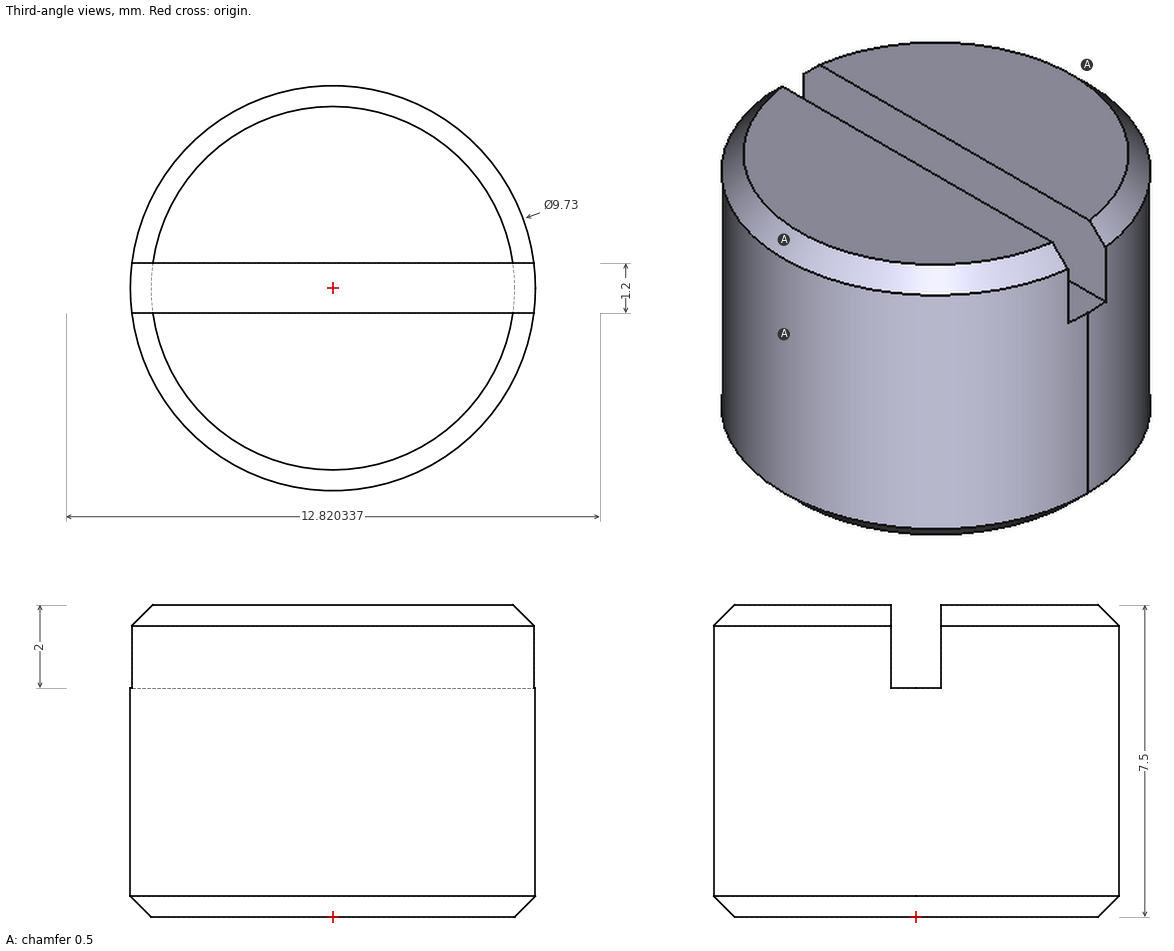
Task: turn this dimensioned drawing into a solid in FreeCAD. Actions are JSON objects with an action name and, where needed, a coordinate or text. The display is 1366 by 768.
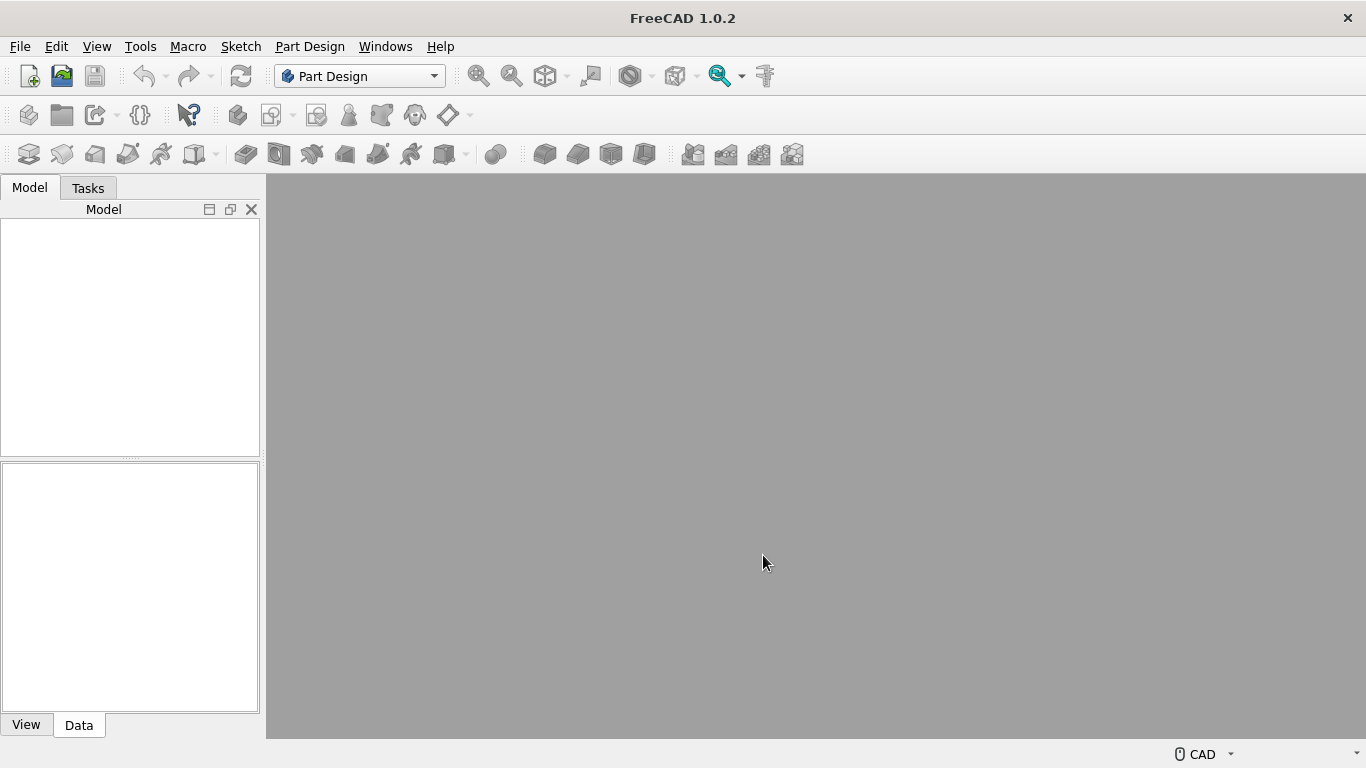
{"action": "left_click", "coordinate": [29, 76]}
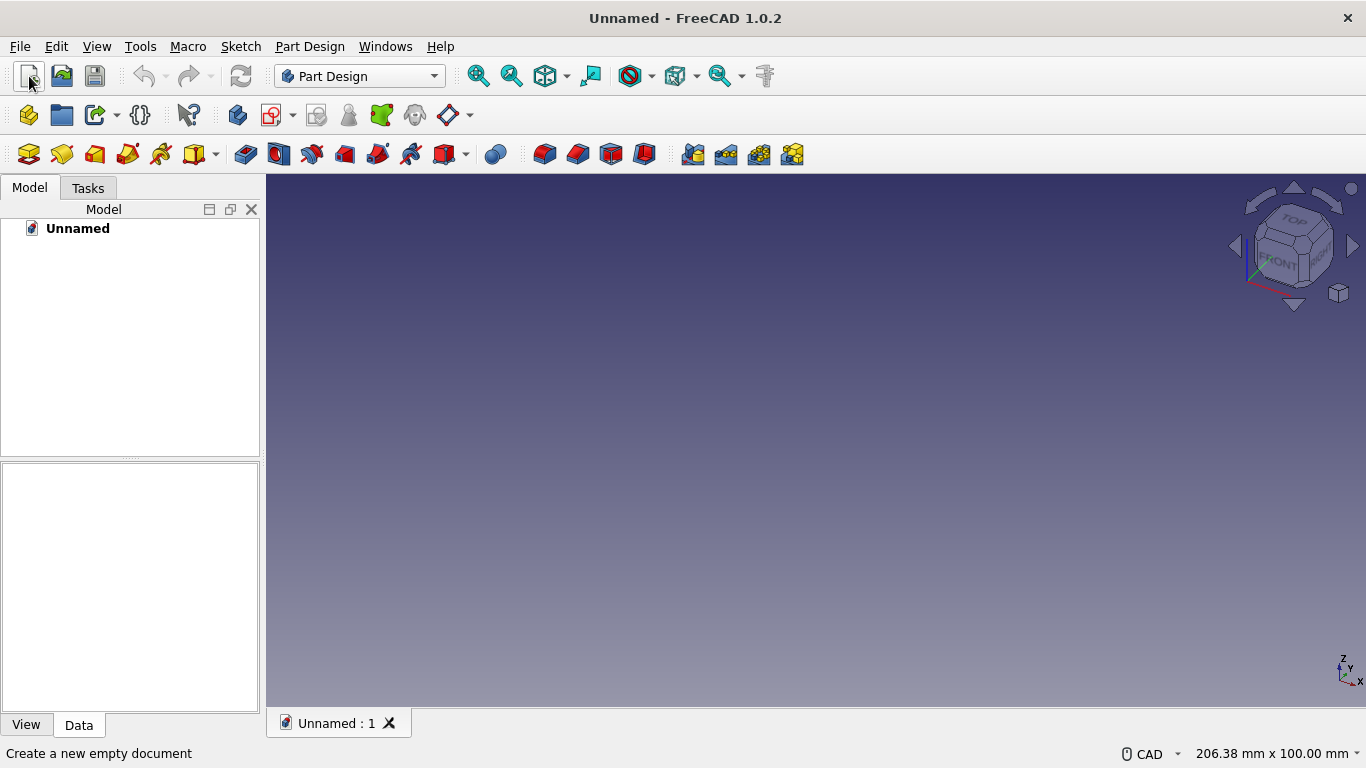
{"action": "left_click", "coordinate": [270, 116]}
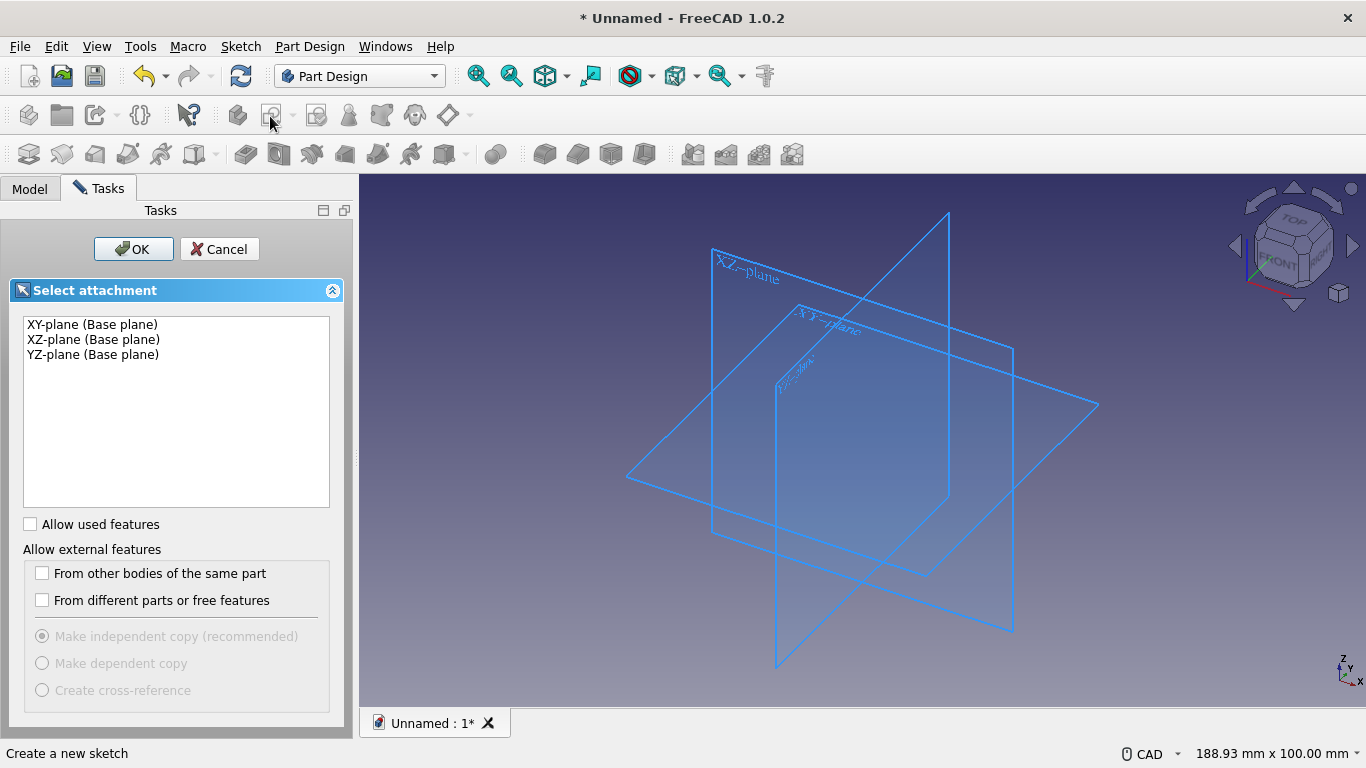
{"action": "left_click", "coordinate": [84, 324]}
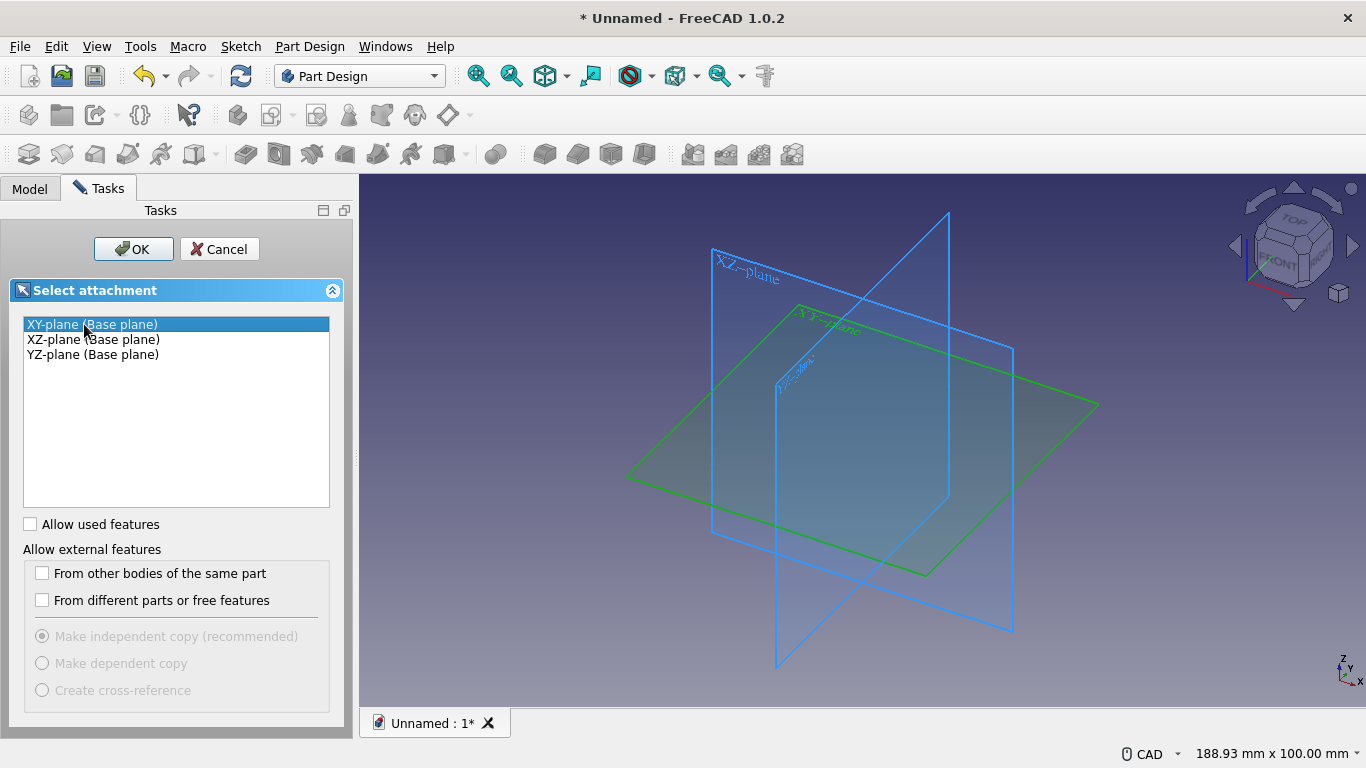
{"action": "left_click", "coordinate": [134, 249]}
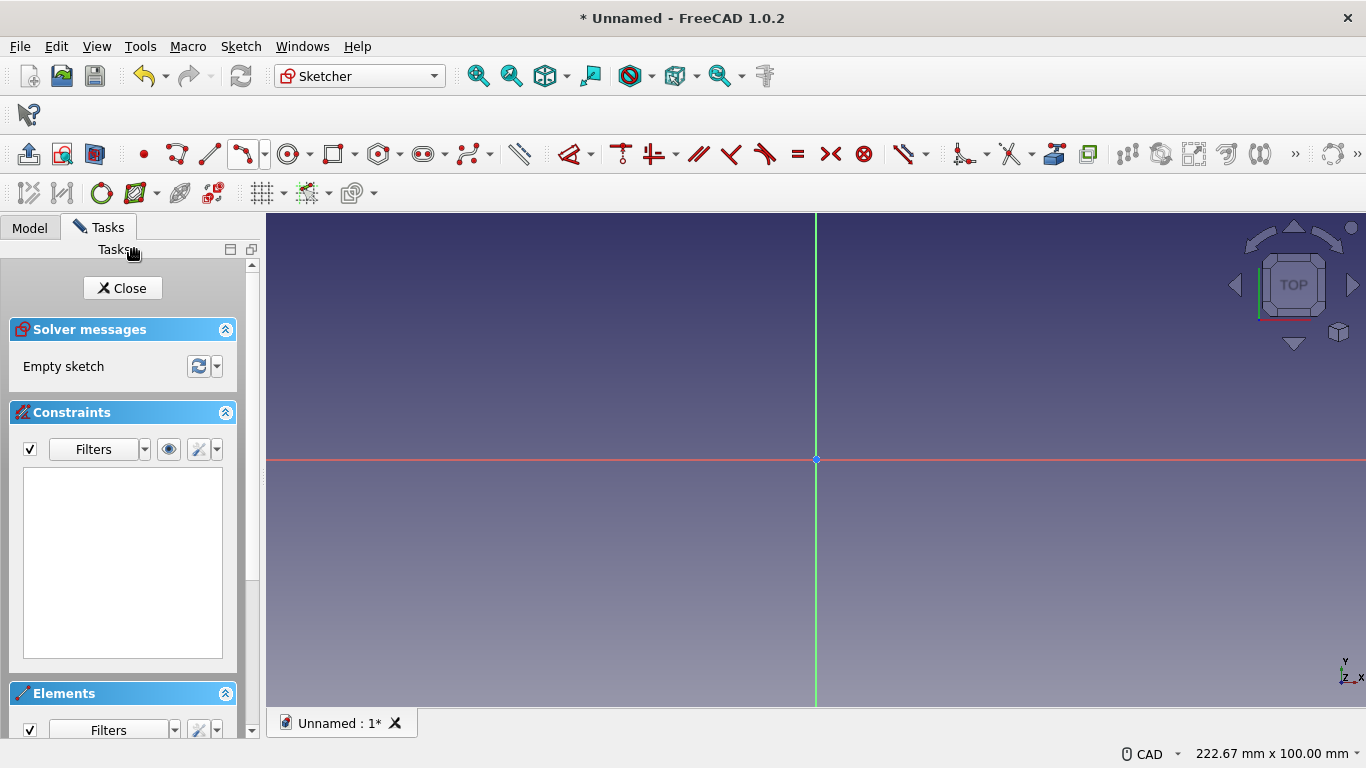
{"action": "scroll", "coordinate": [830, 460], "scroll_direction": "up", "scroll_amount": 9}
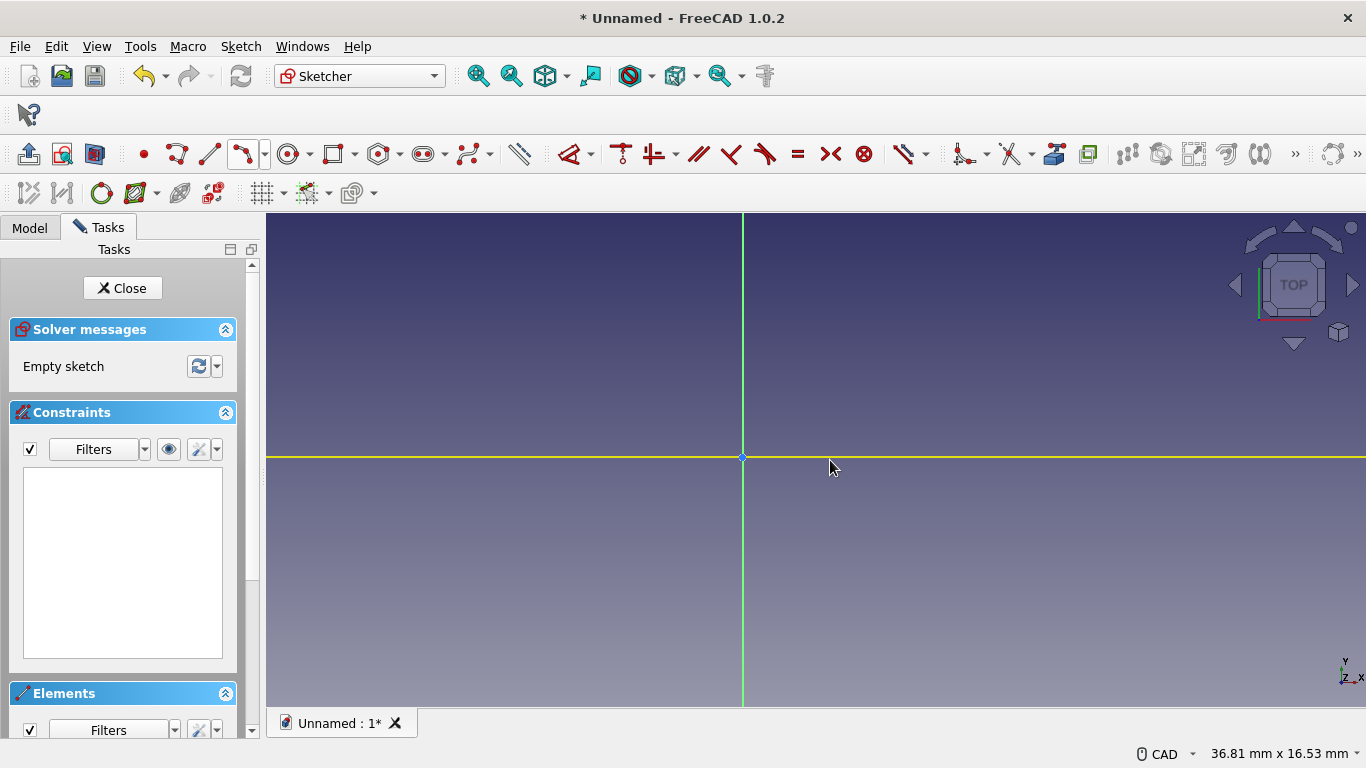
{"action": "left_click", "coordinate": [288, 154]}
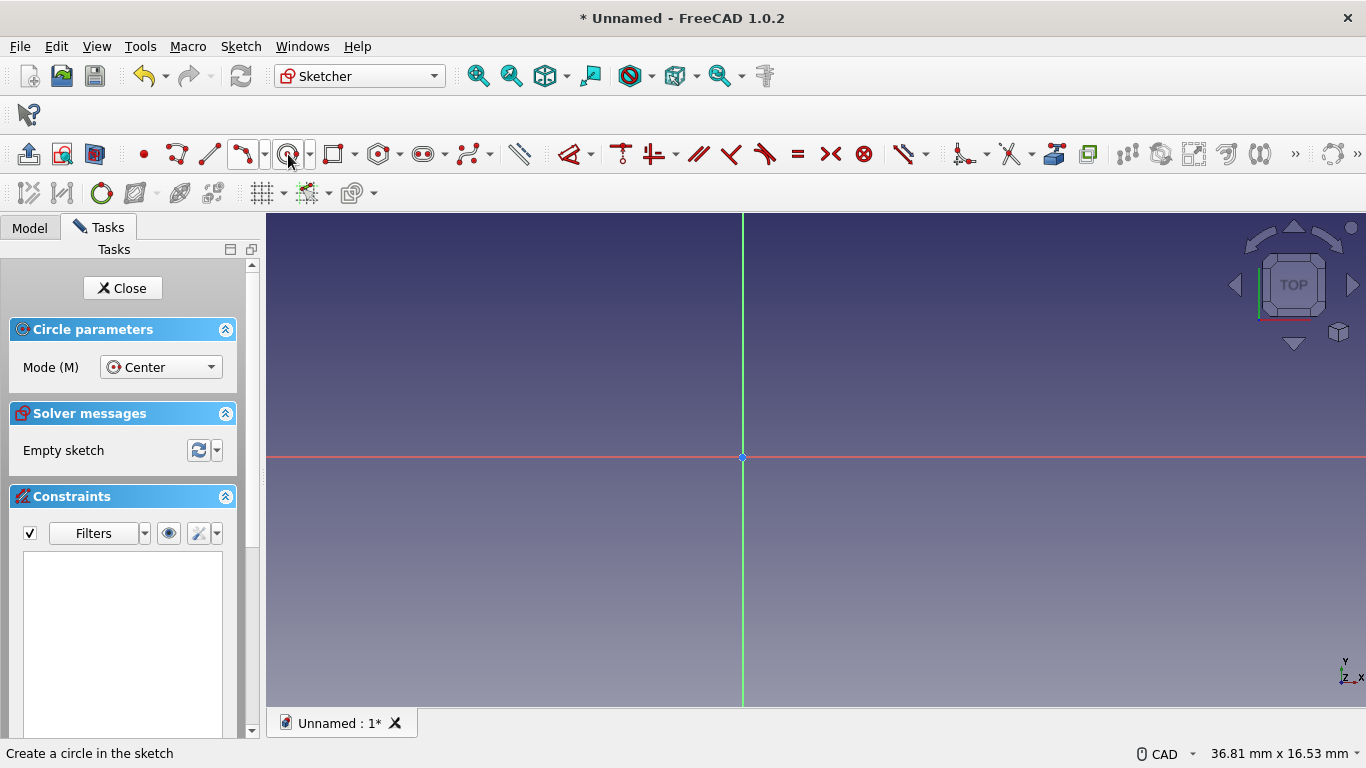
{"action": "left_click", "coordinate": [743, 457]}
{"action": "left_click", "coordinate": [846, 355]}
{"action": "key", "text": "Escape"}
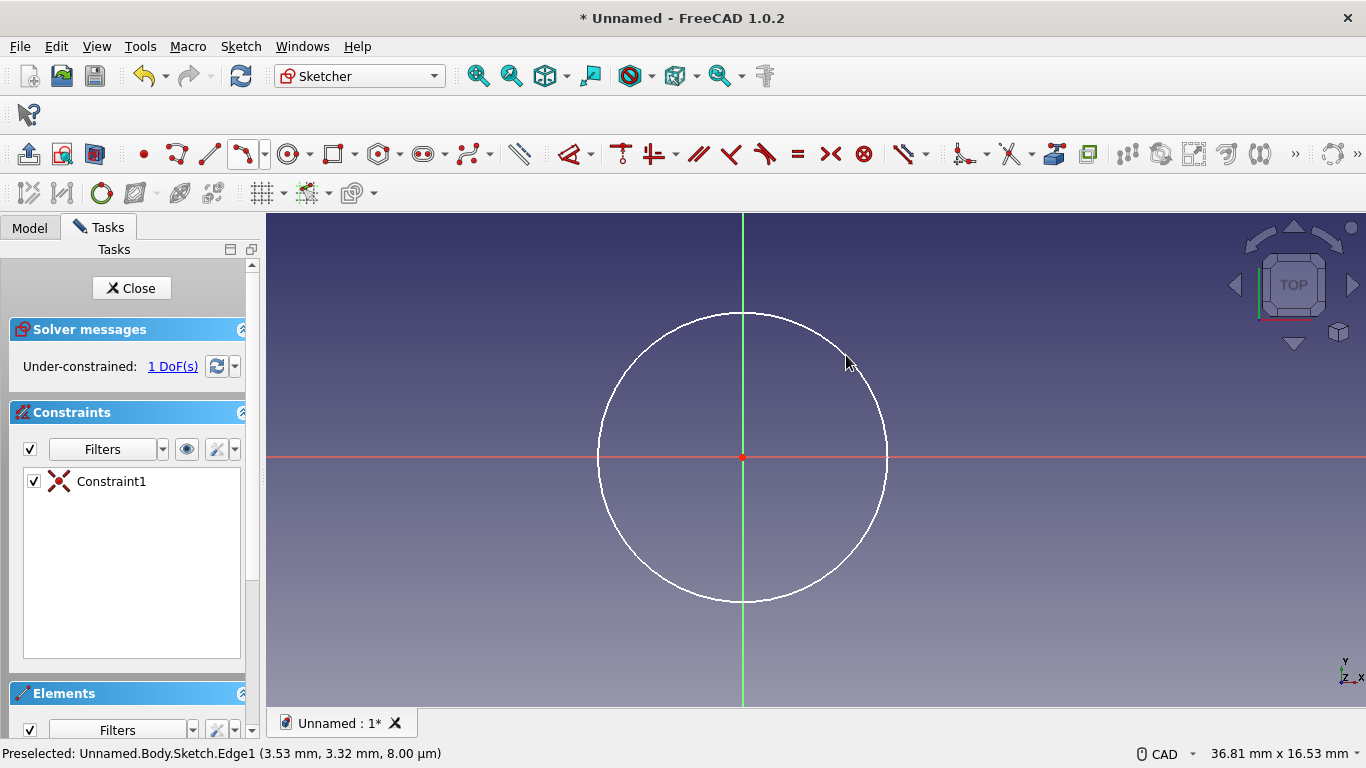
{"action": "left_click", "coordinate": [568, 154]}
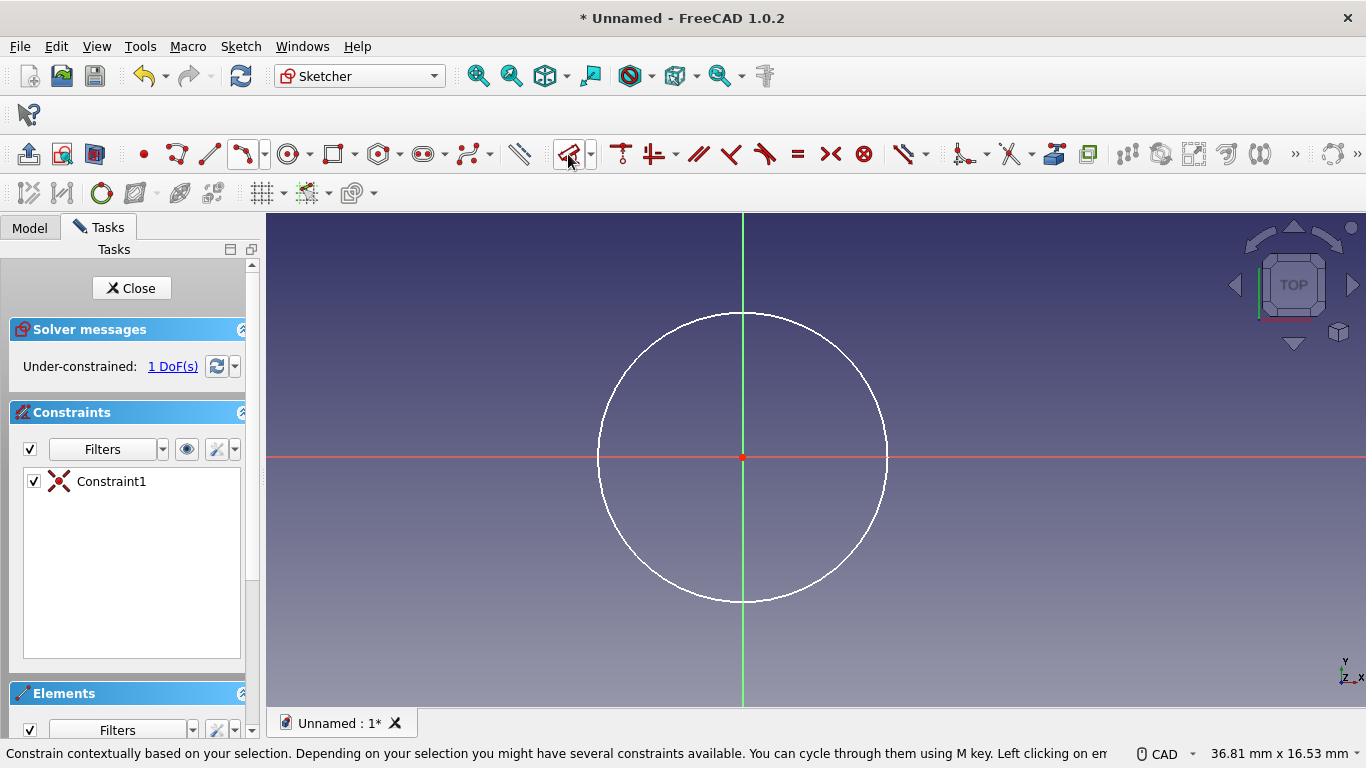
{"action": "left_click", "coordinate": [845, 355]}
{"action": "left_click", "coordinate": [868, 332]}